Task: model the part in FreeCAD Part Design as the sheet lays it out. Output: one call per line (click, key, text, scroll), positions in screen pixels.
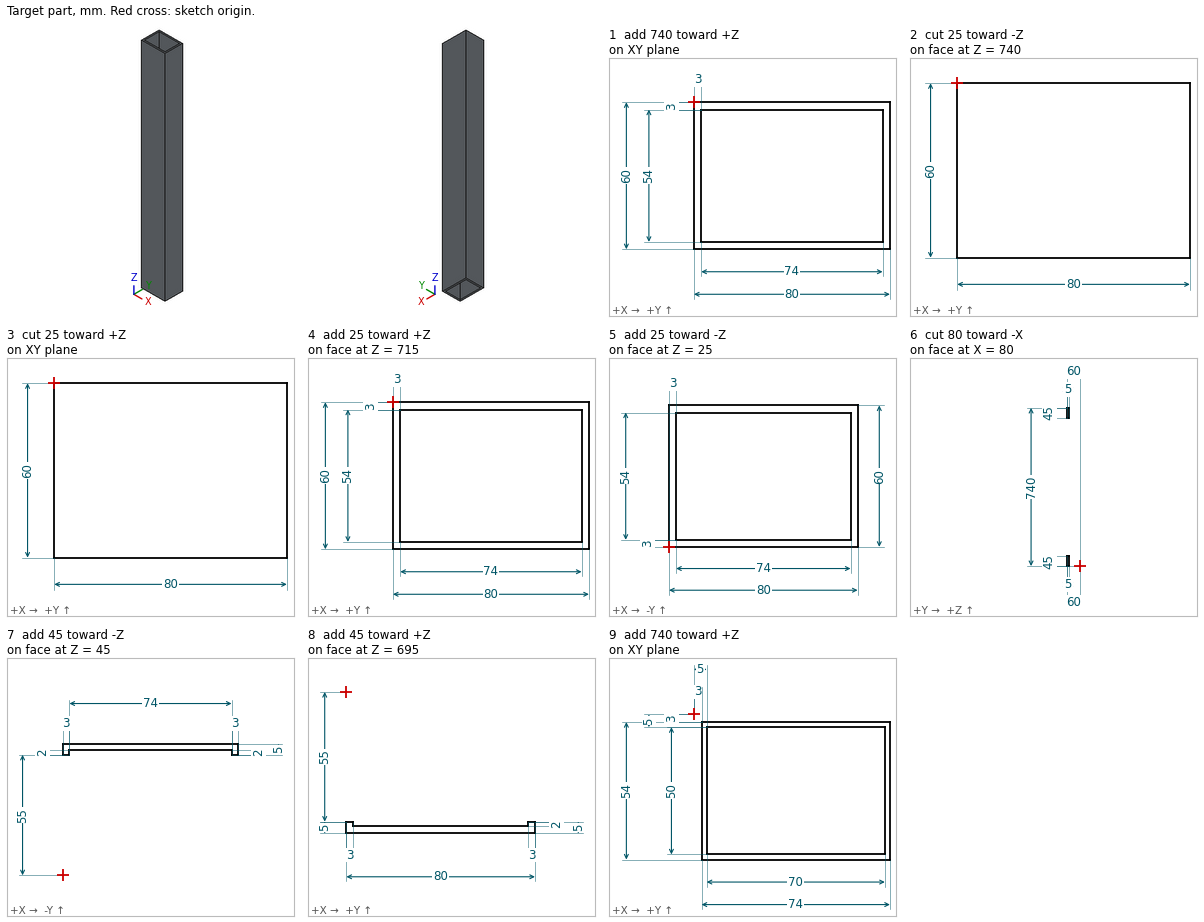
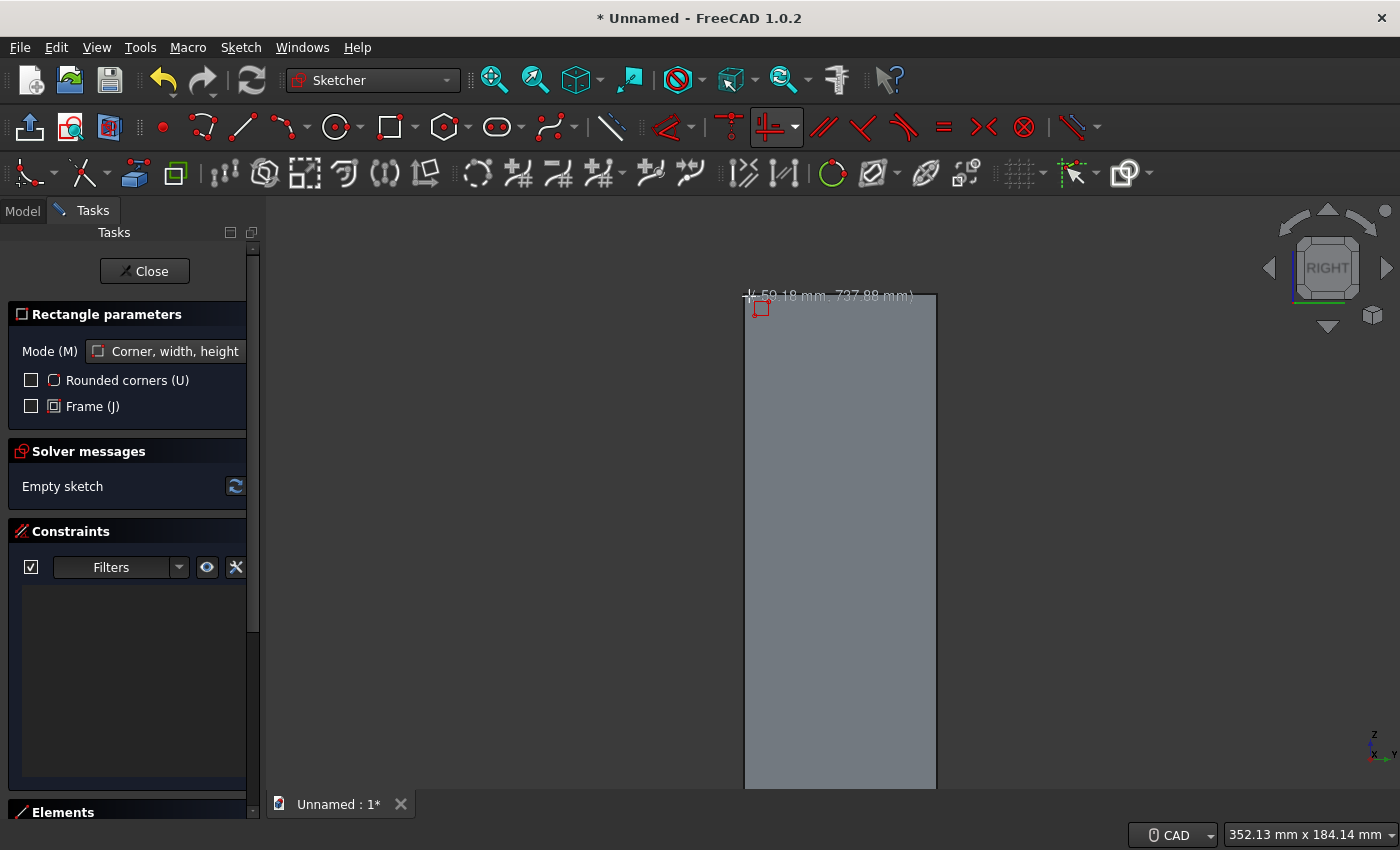
scroll(749, 296, down, 9)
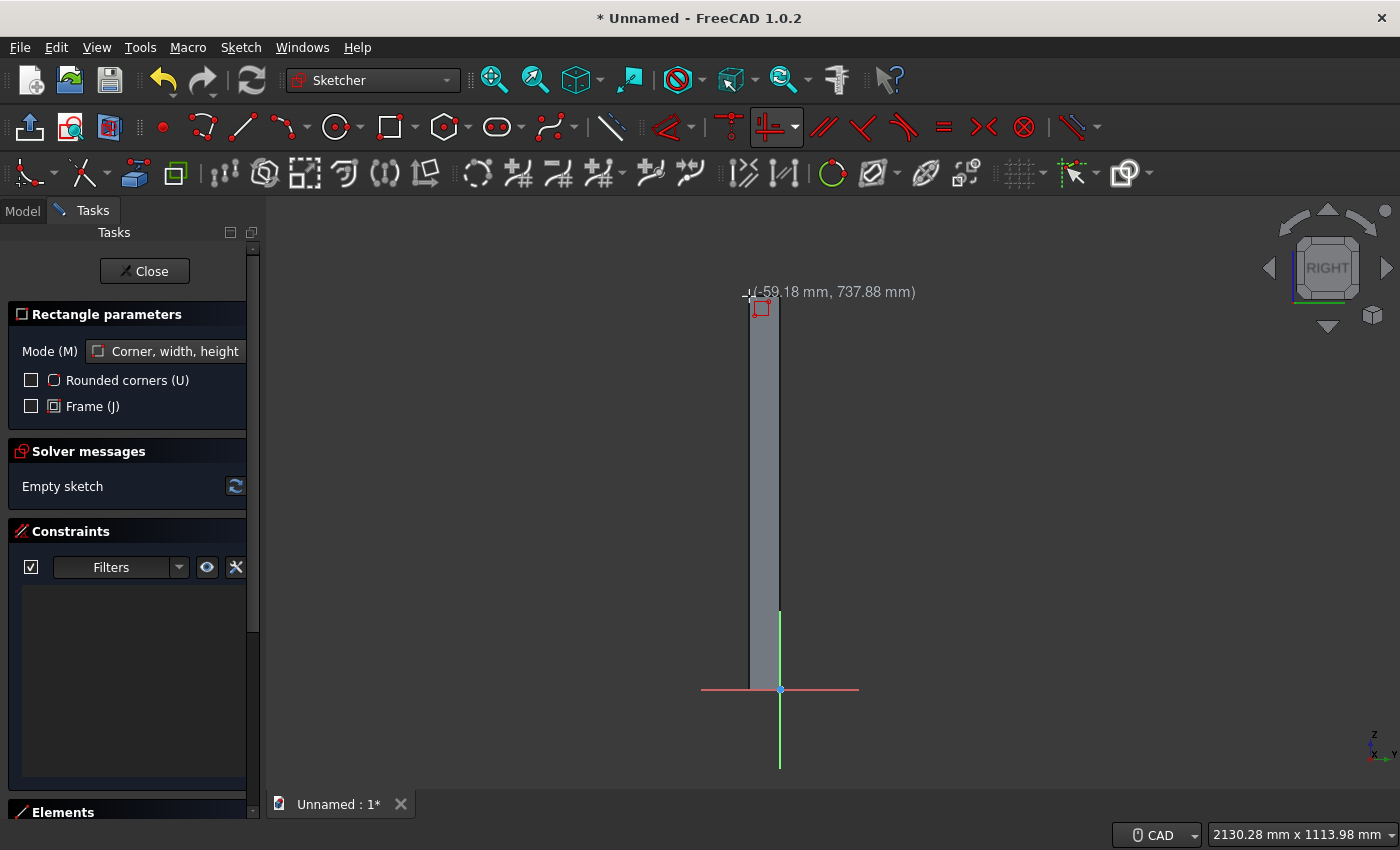
click(749, 296)
click(751, 320)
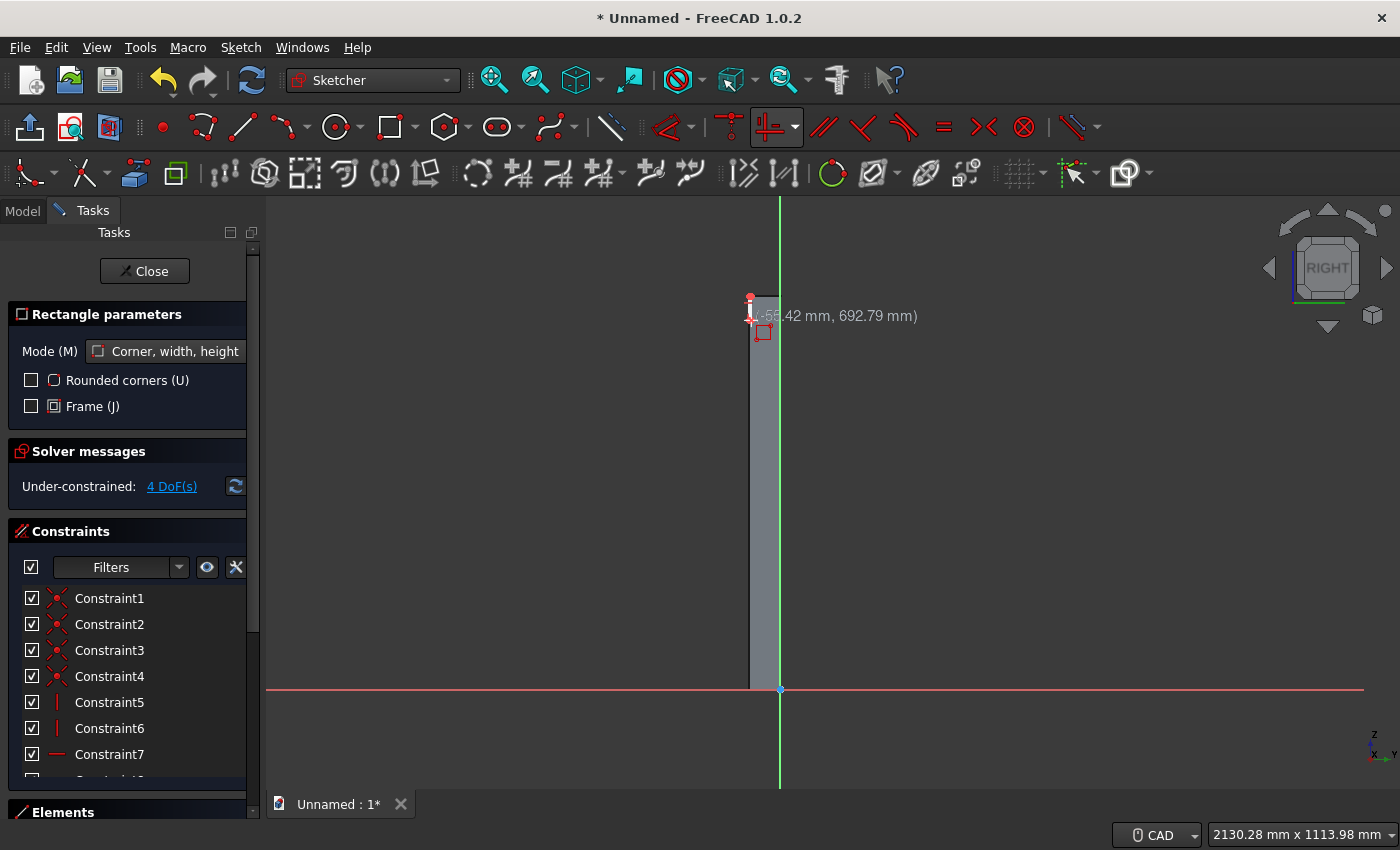
scroll(749, 666, up, 9)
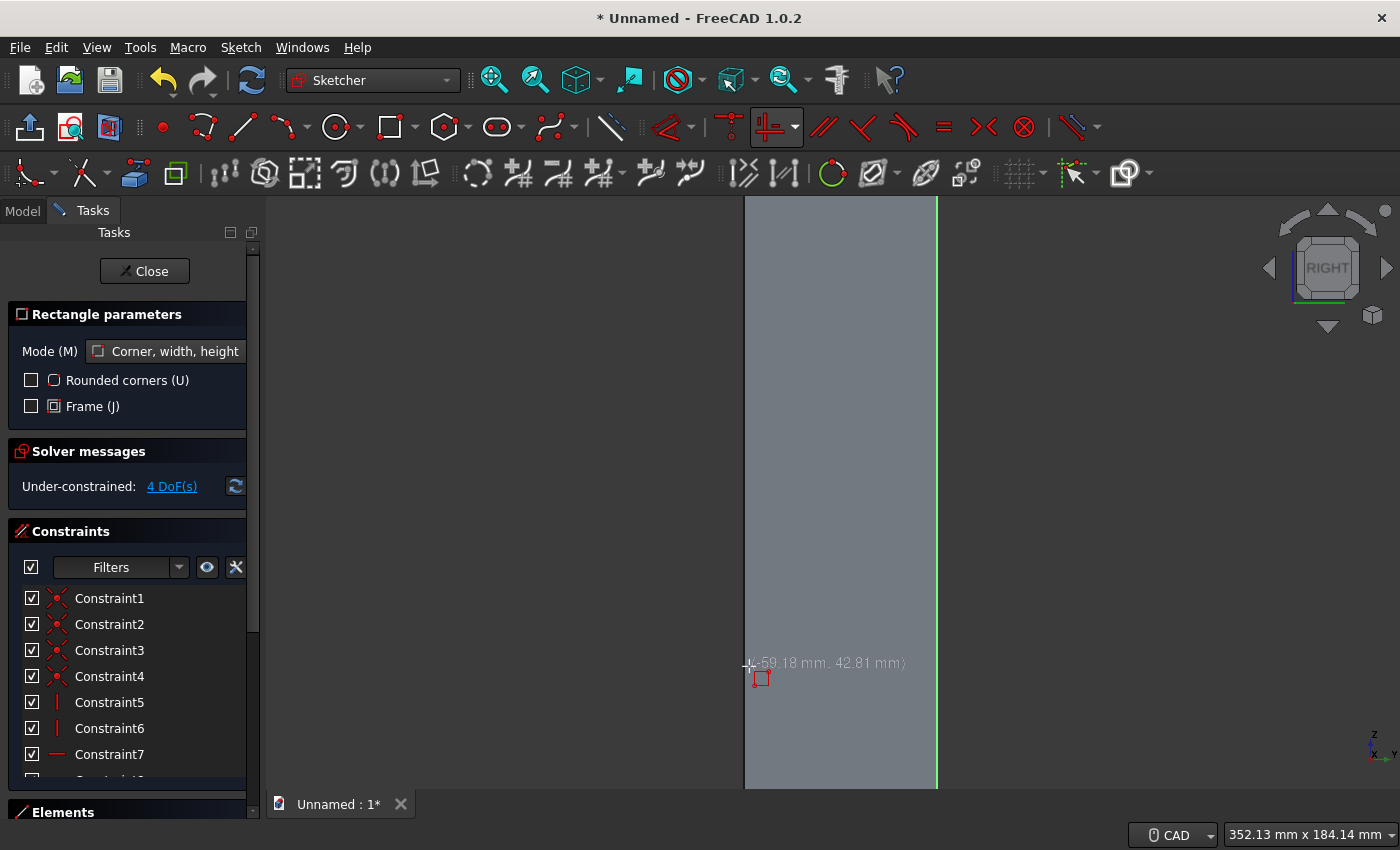
scroll(749, 666, down, 9)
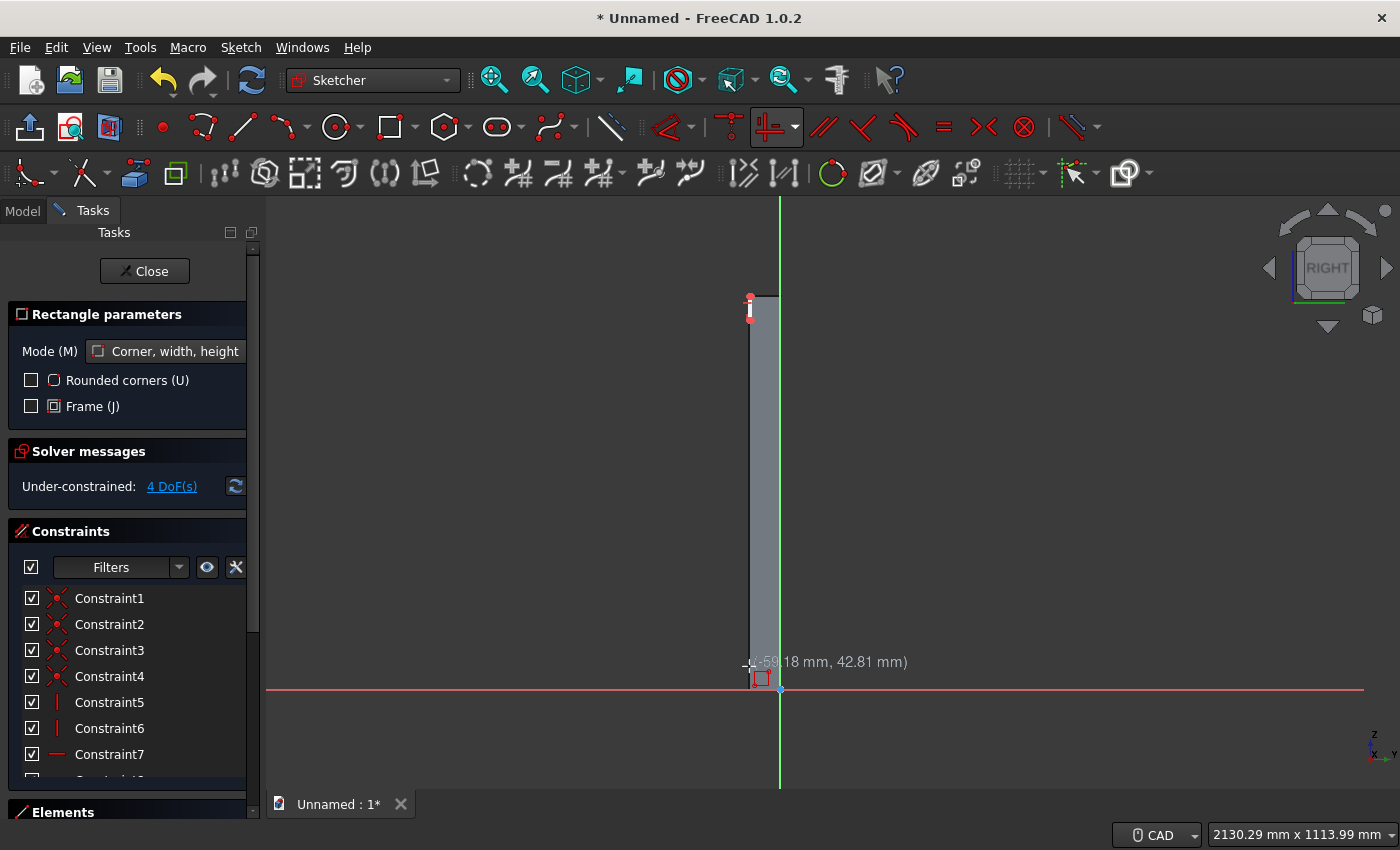
click(749, 666)
click(751, 690)
key(Escape)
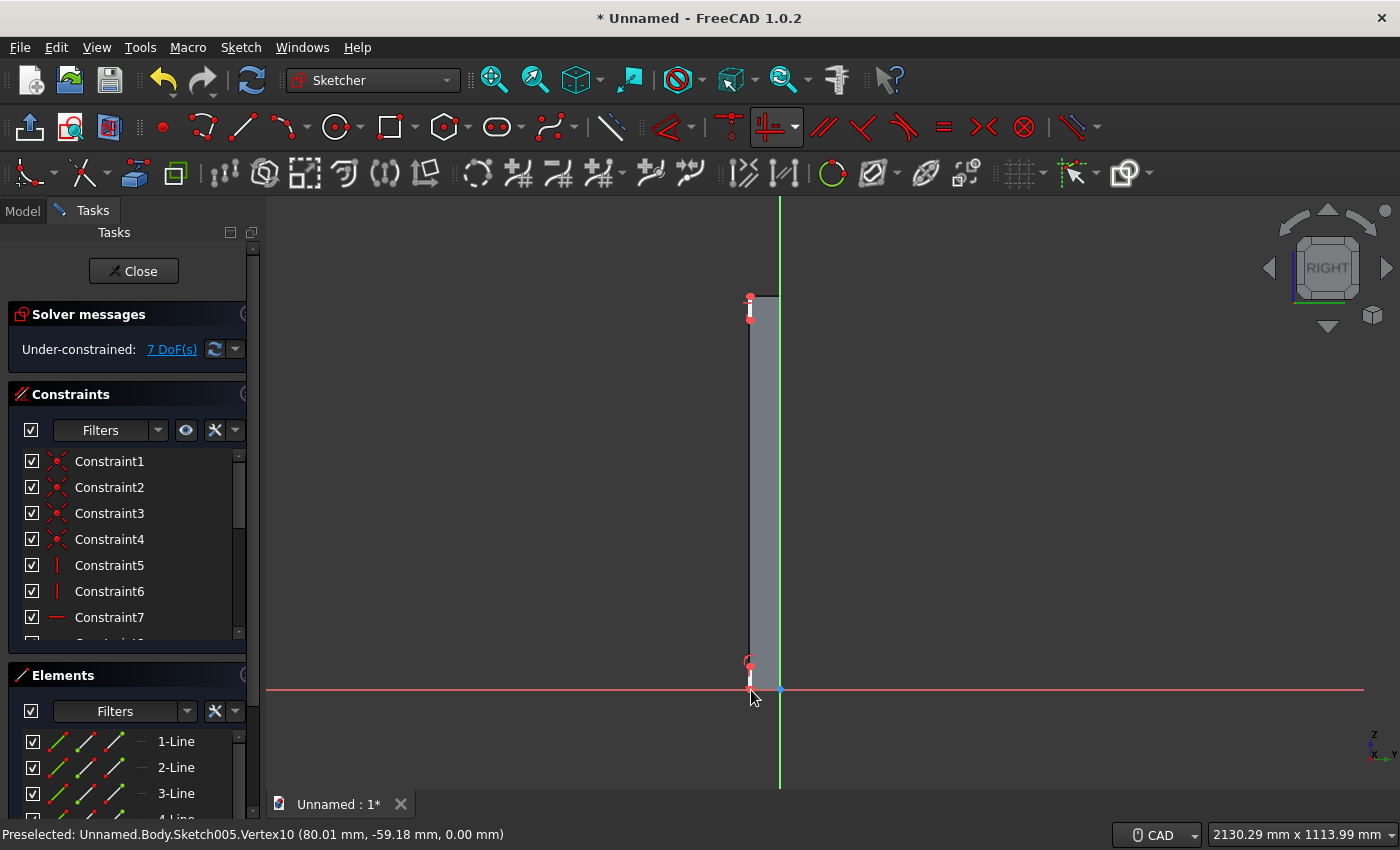
key(d)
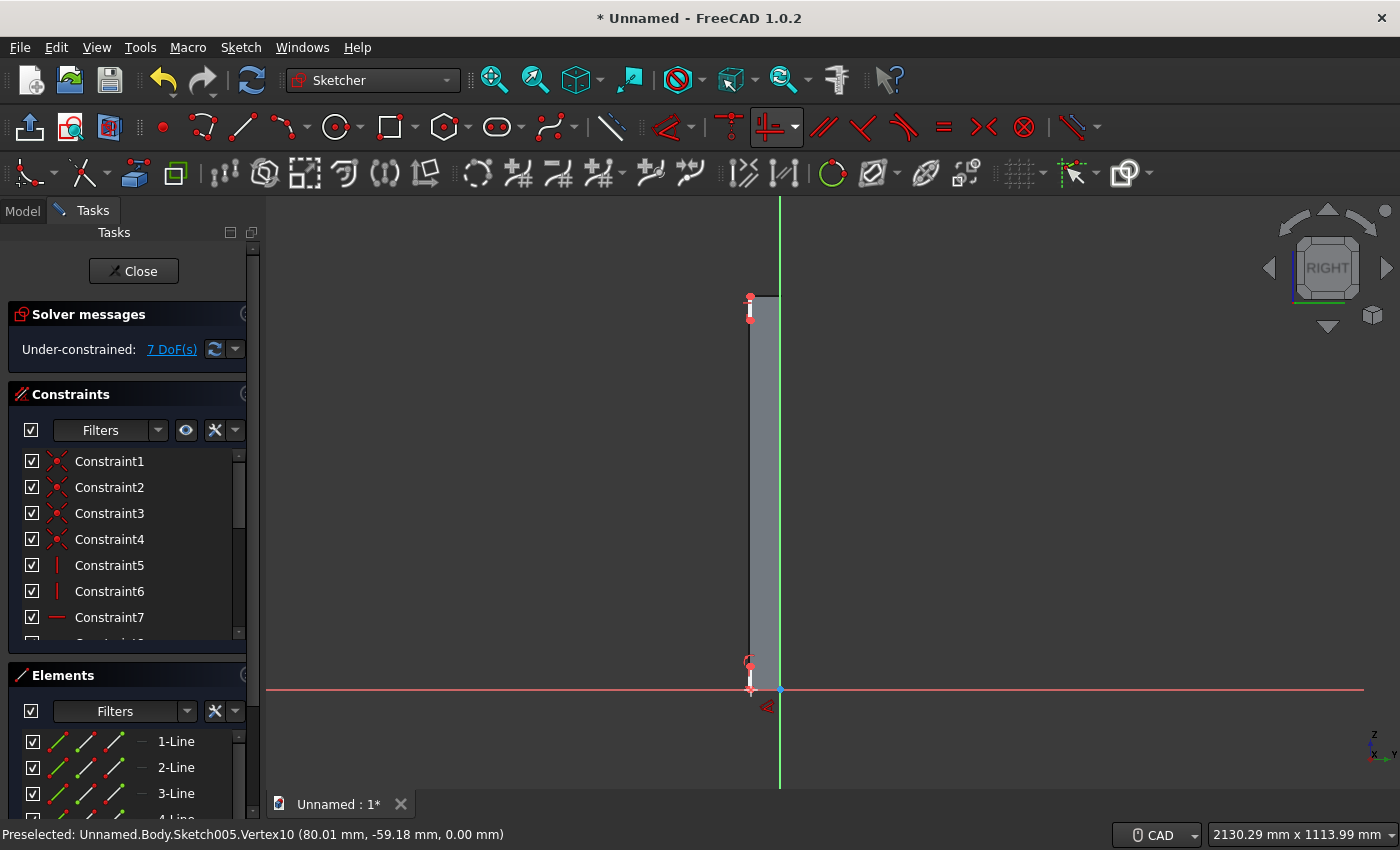
scroll(750, 321, up, 14)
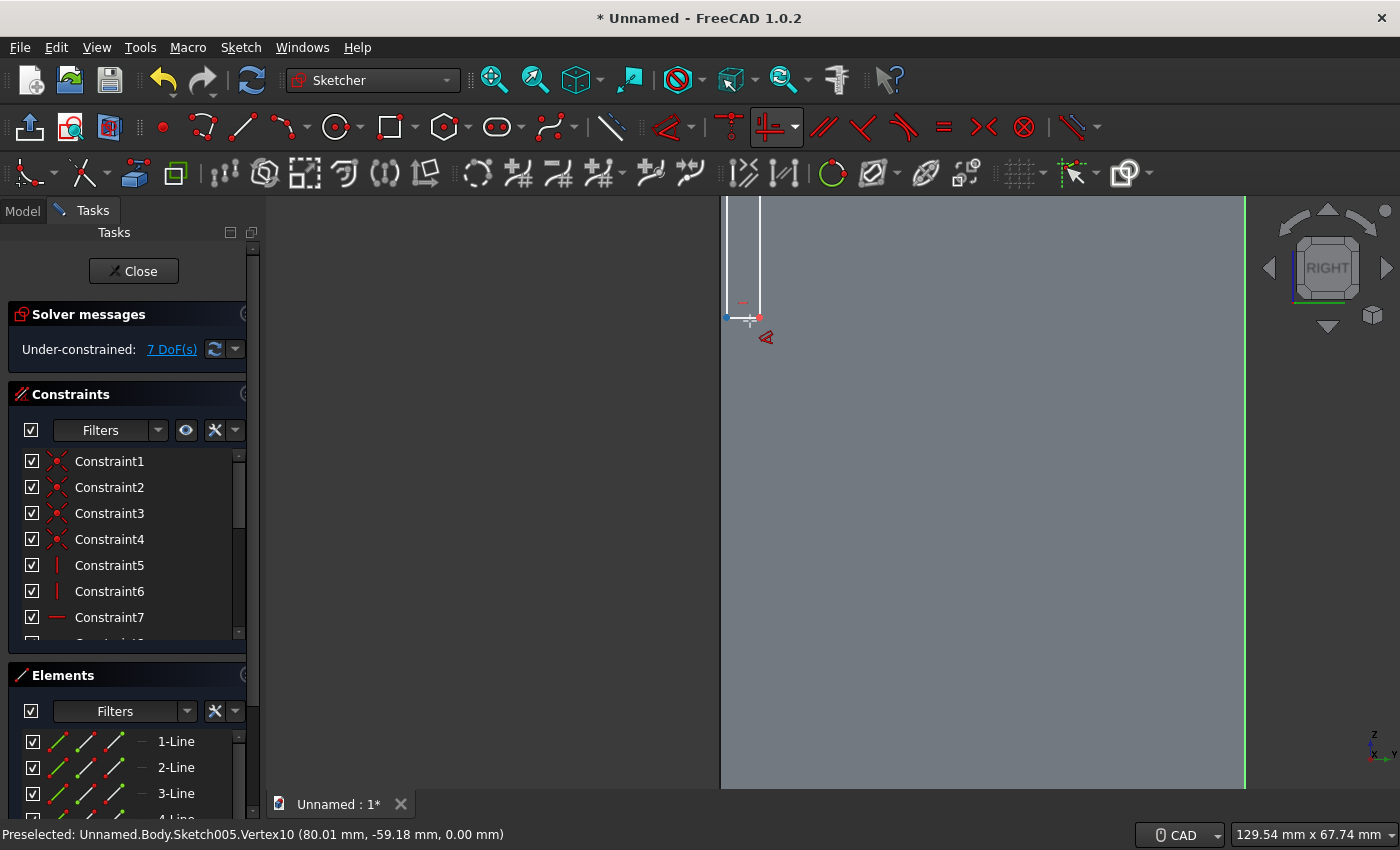
click(743, 318)
click(743, 284)